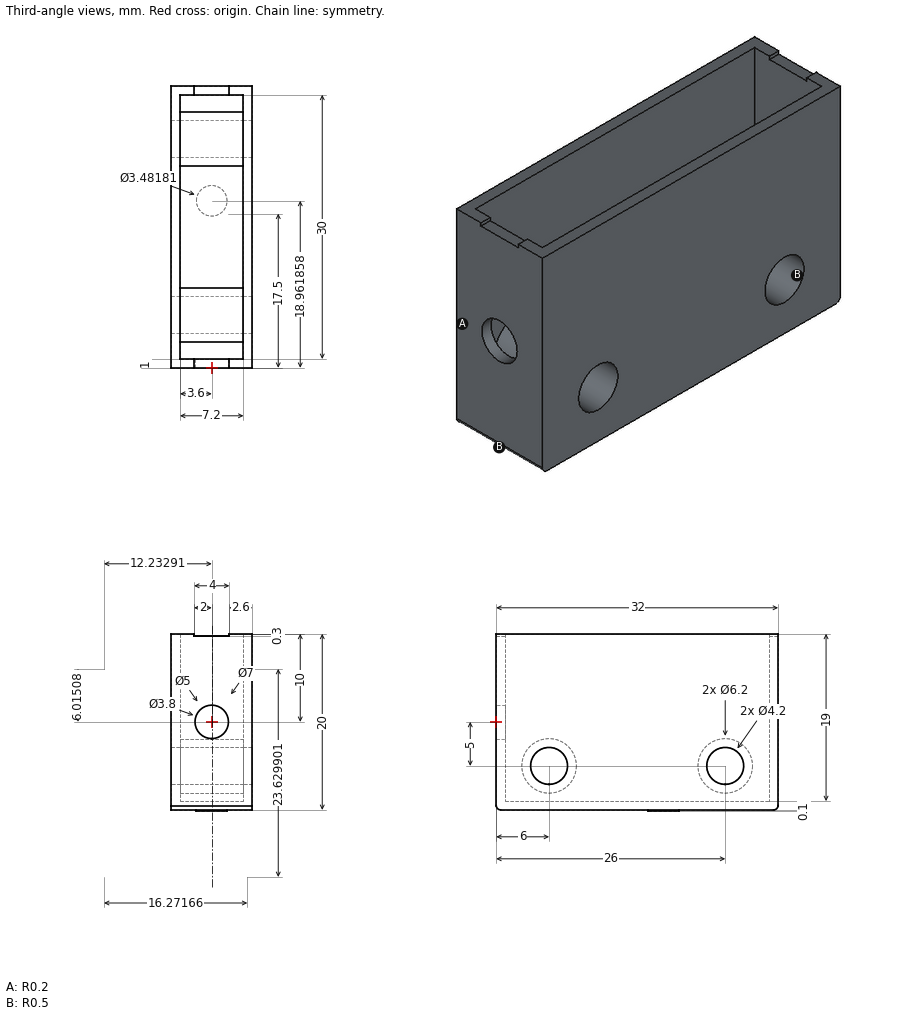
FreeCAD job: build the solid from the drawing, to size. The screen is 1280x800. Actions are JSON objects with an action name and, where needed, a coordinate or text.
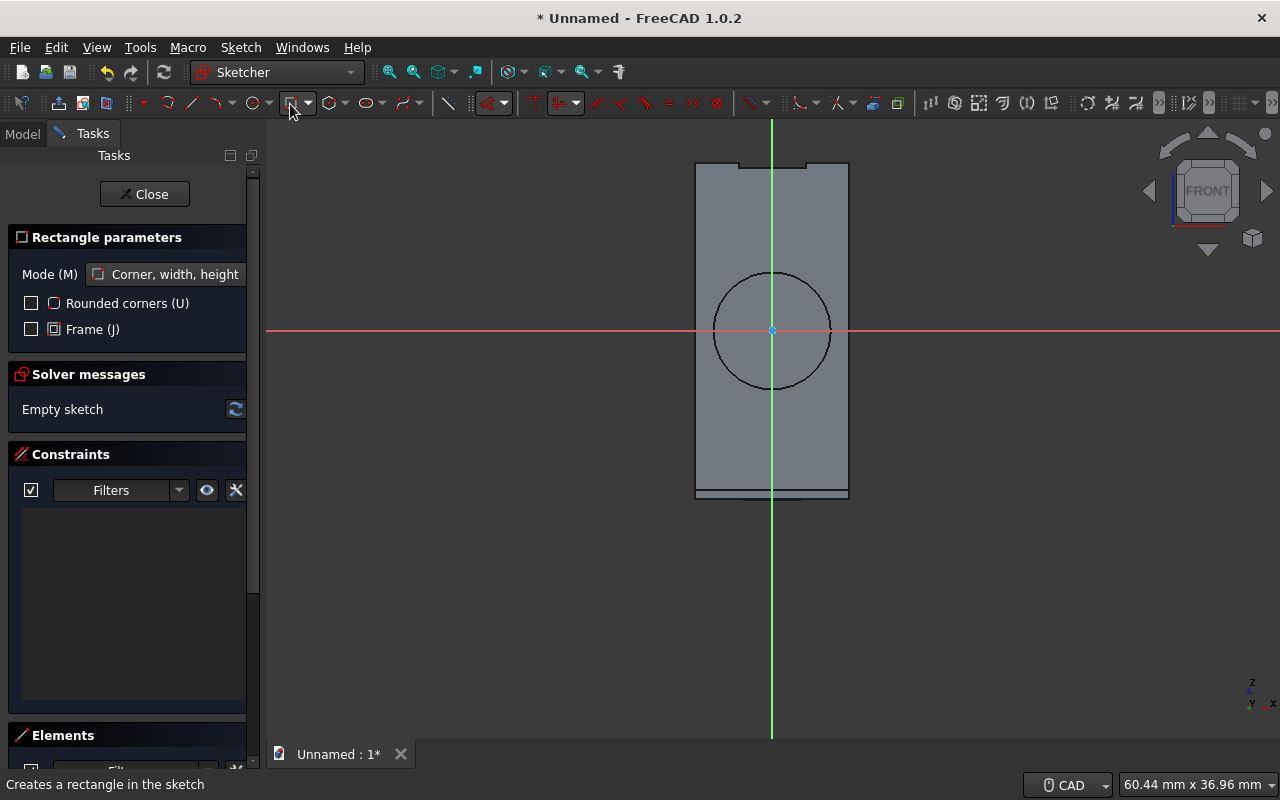
{"action": "left_click", "coordinate": [567, 230]}
{"action": "mouse_move", "coordinate": [840, 626]}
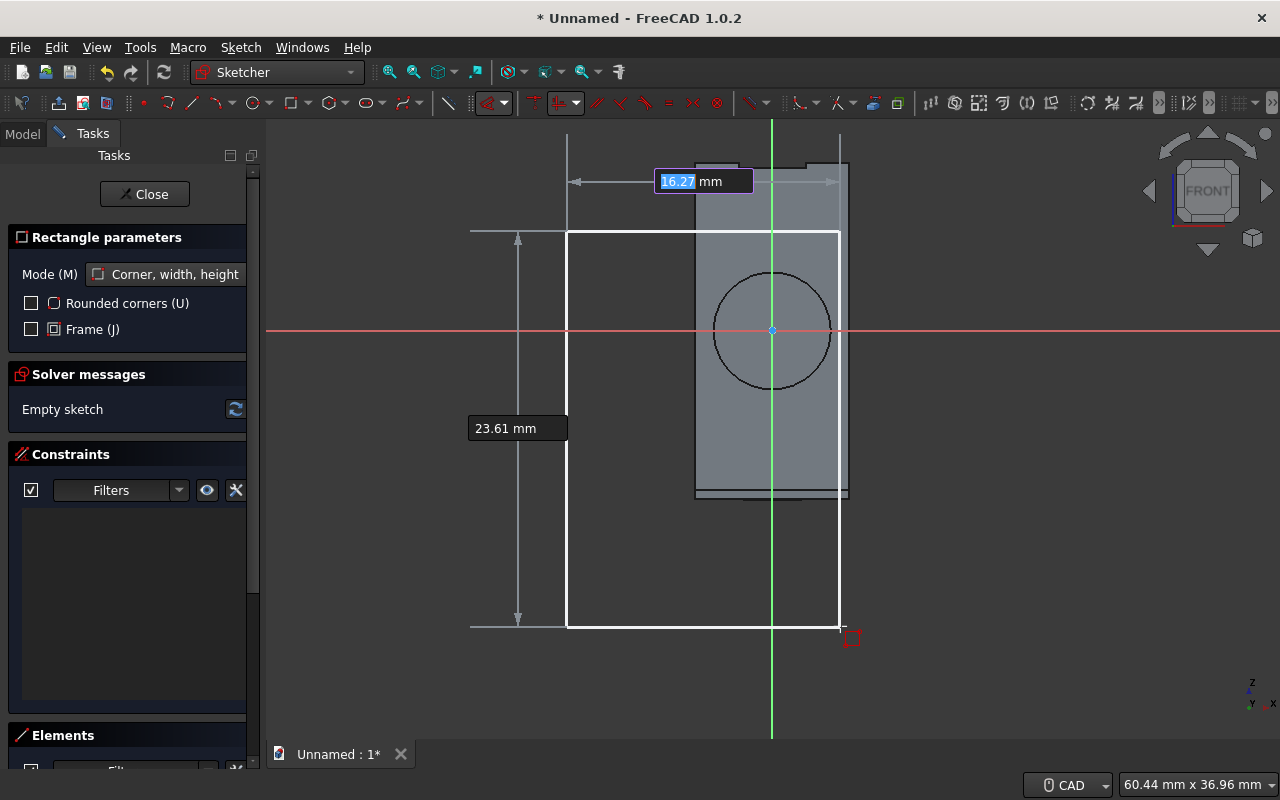
{"action": "type", "text": "16.27166"}
{"action": "key", "text": "Tab"}
{"action": "type", "text": "23.629901"}
{"action": "key", "text": "Return"}
{"action": "key", "text": "Escape"}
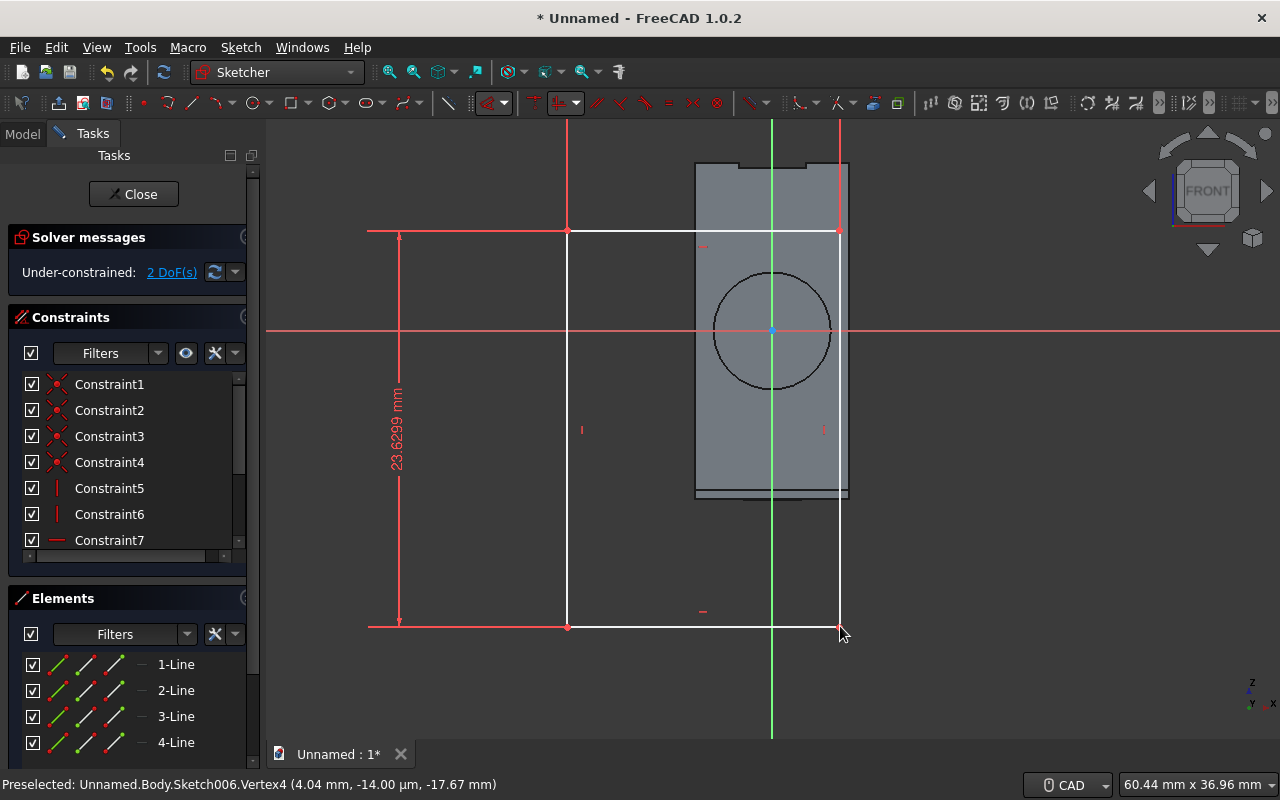
{"action": "left_click", "coordinate": [567, 231]}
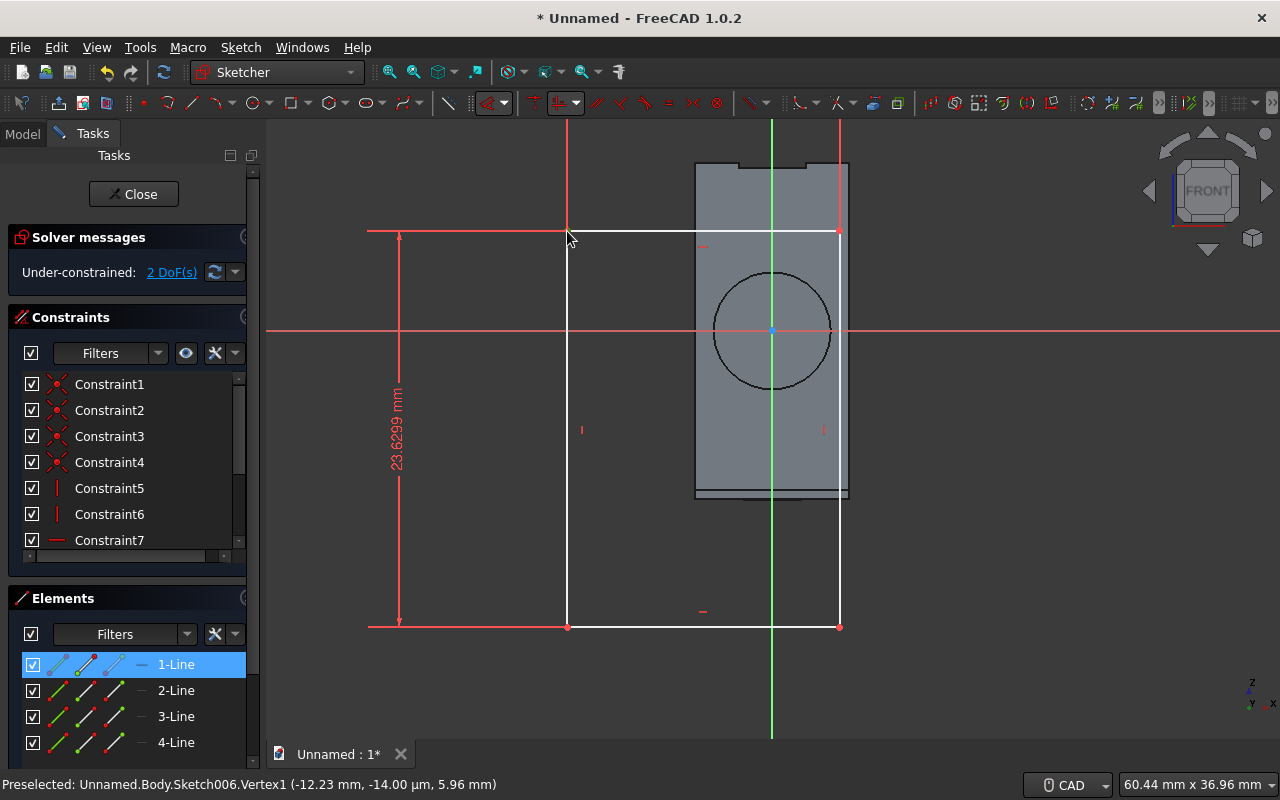
{"action": "key", "text": "i"}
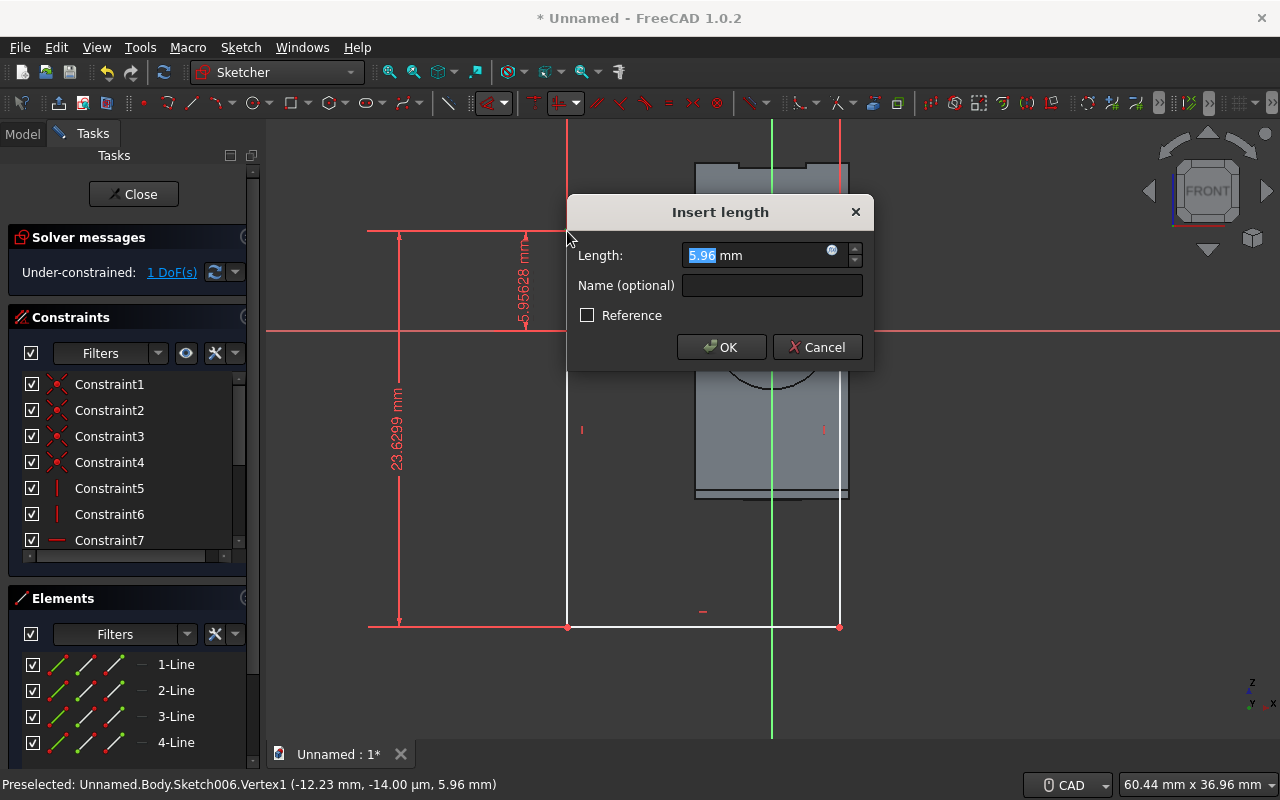
{"action": "type", "text": "6.01508"}
{"action": "key", "text": "Return"}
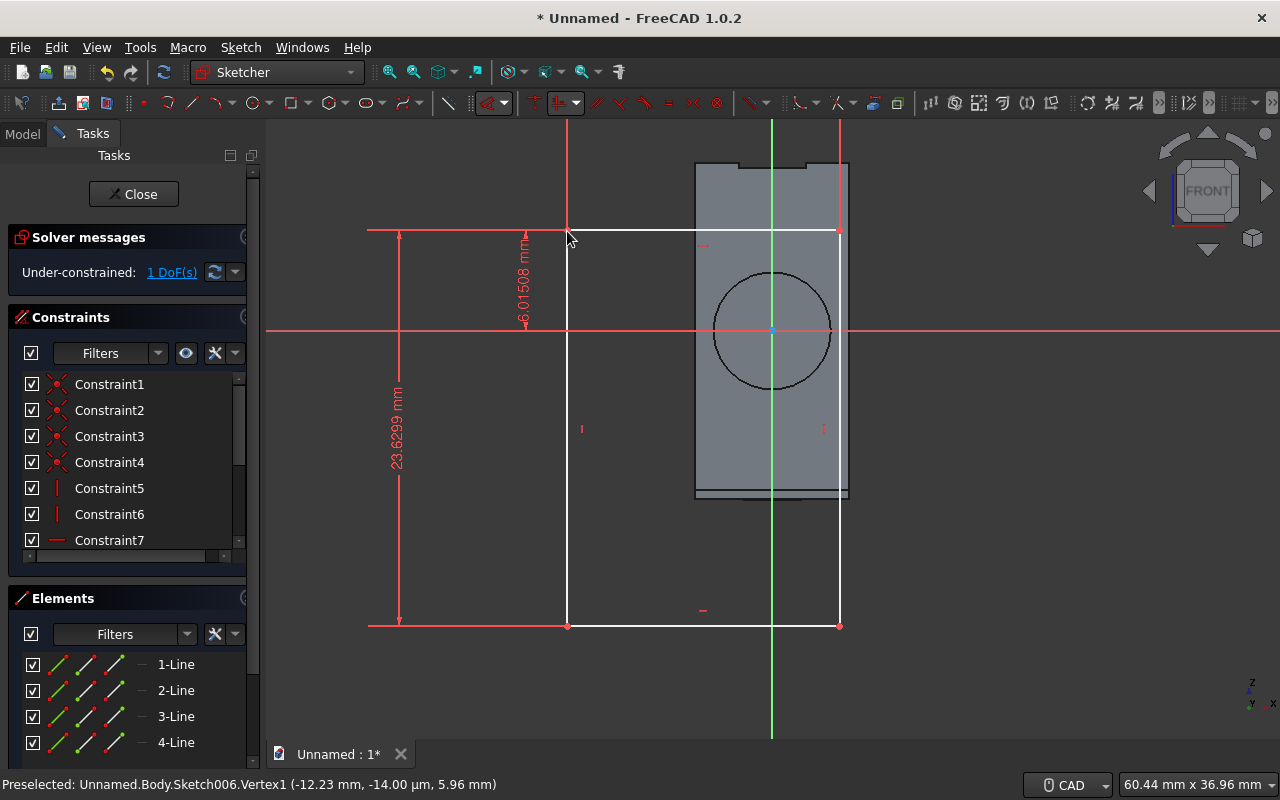
{"action": "left_click", "coordinate": [567, 230]}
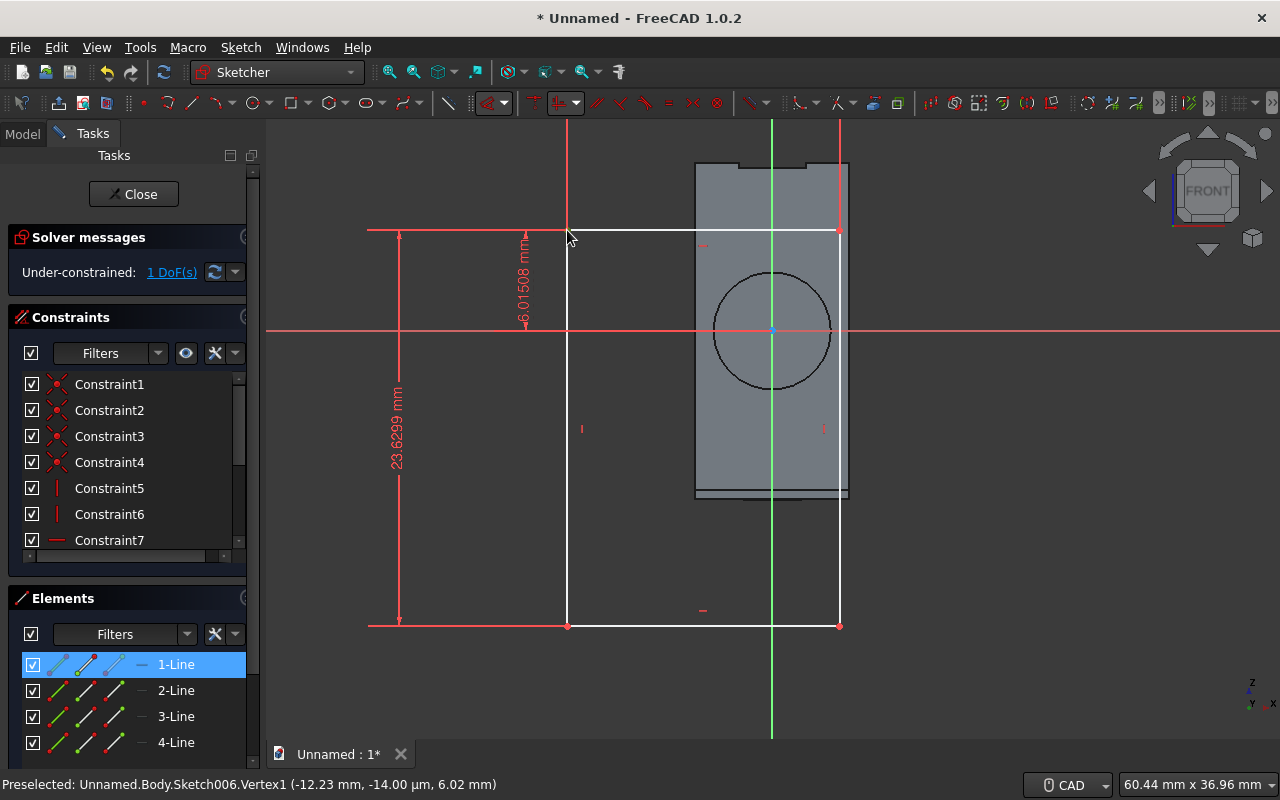
{"action": "left_click", "coordinate": [506, 104]}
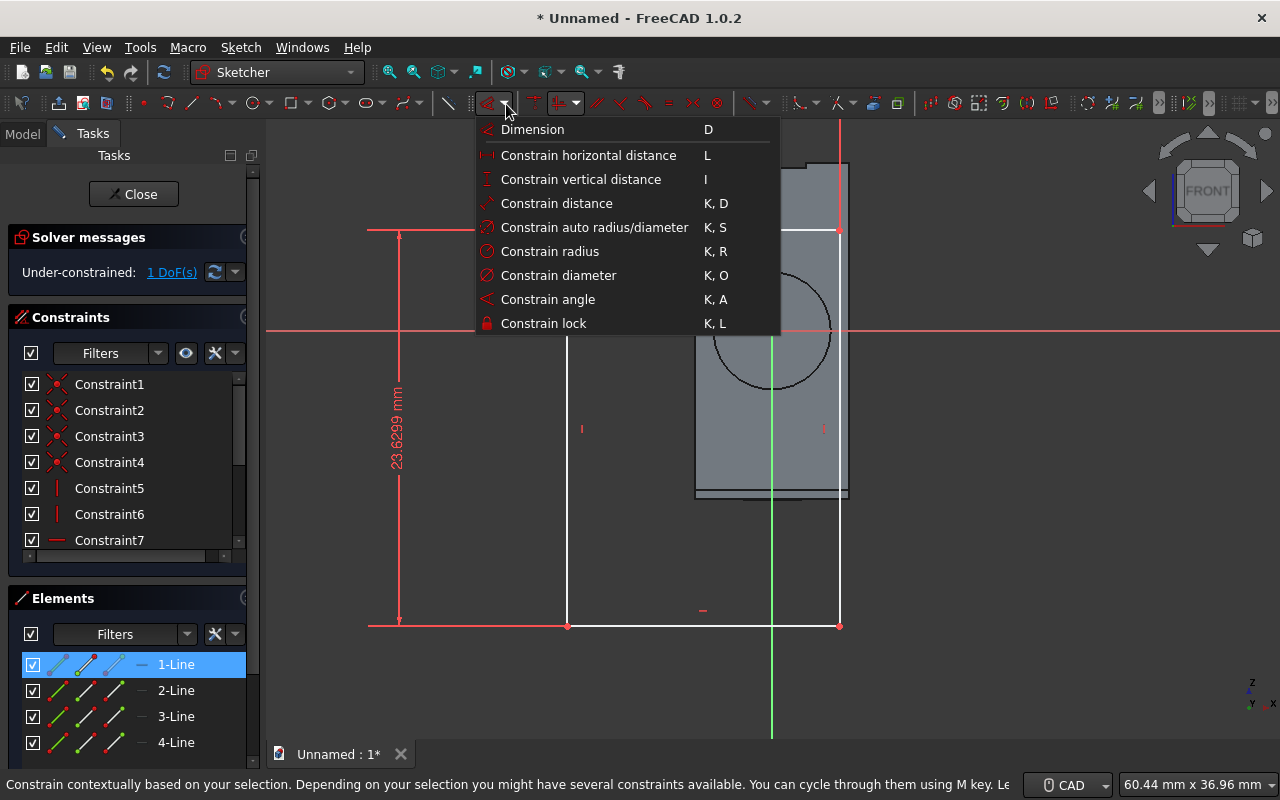
{"action": "left_click", "coordinate": [628, 155]}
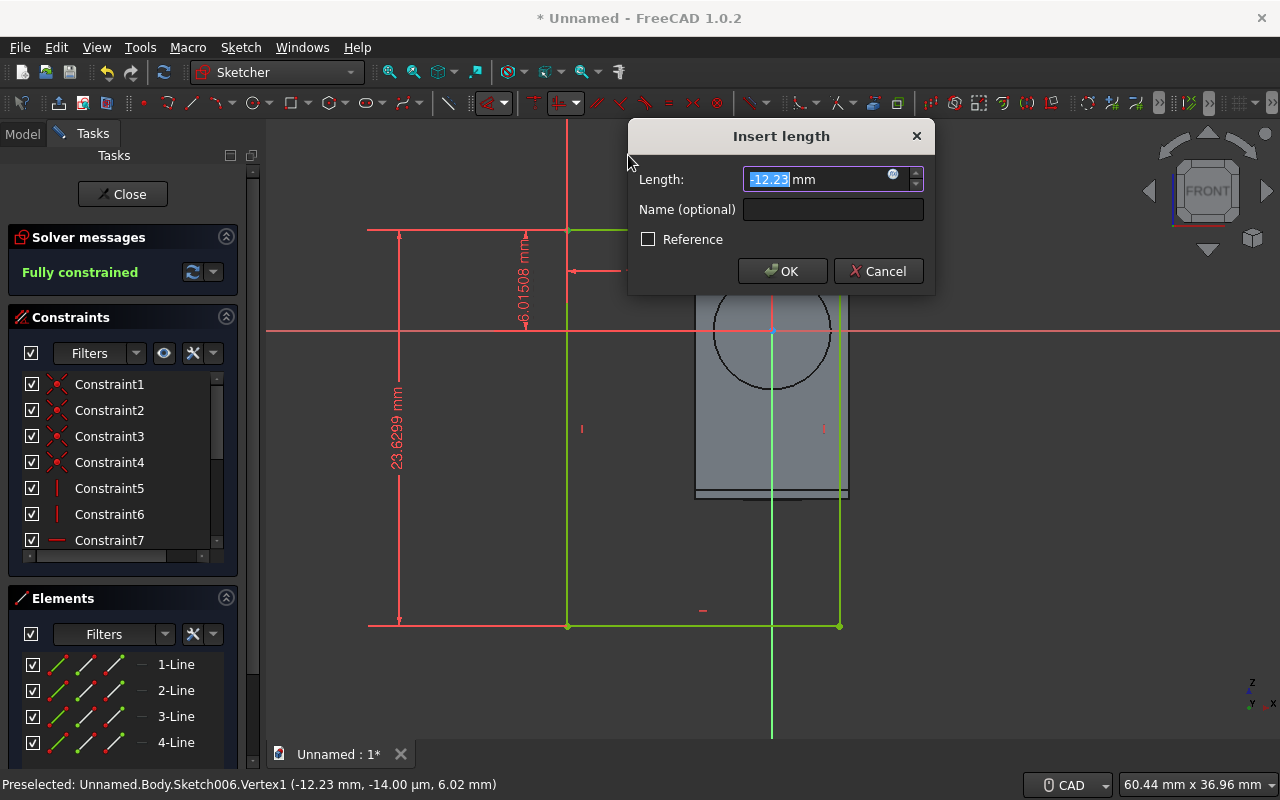
{"action": "type", "text": "-12.23291"}
{"action": "key", "text": "Return"}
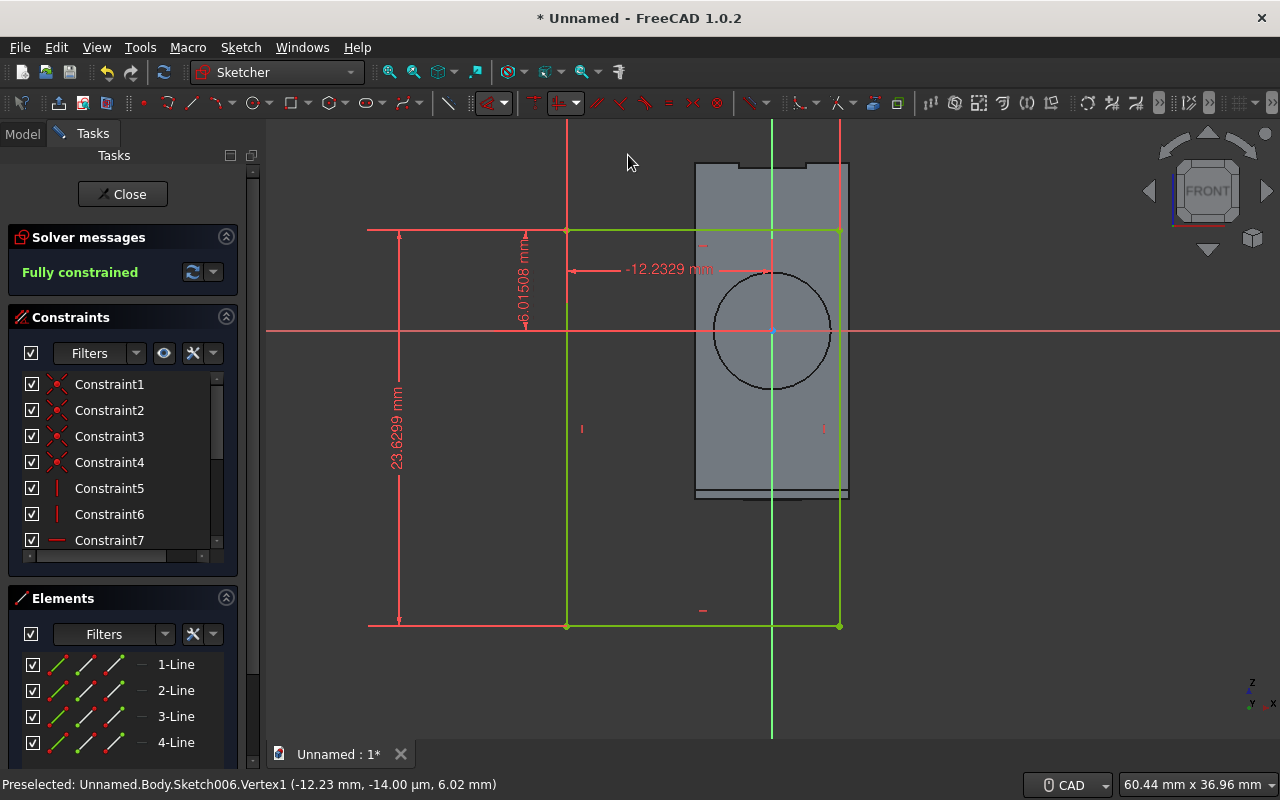
{"action": "left_click", "coordinate": [123, 194]}